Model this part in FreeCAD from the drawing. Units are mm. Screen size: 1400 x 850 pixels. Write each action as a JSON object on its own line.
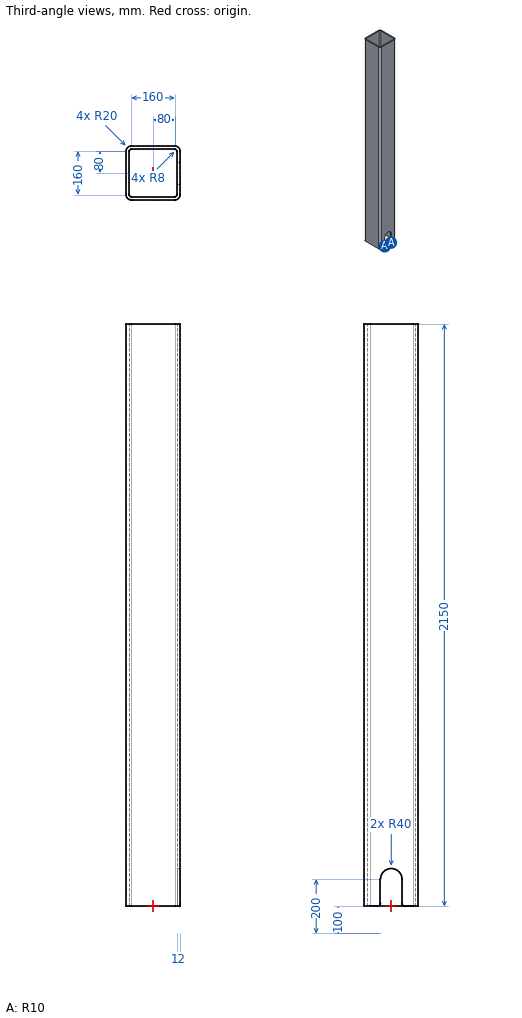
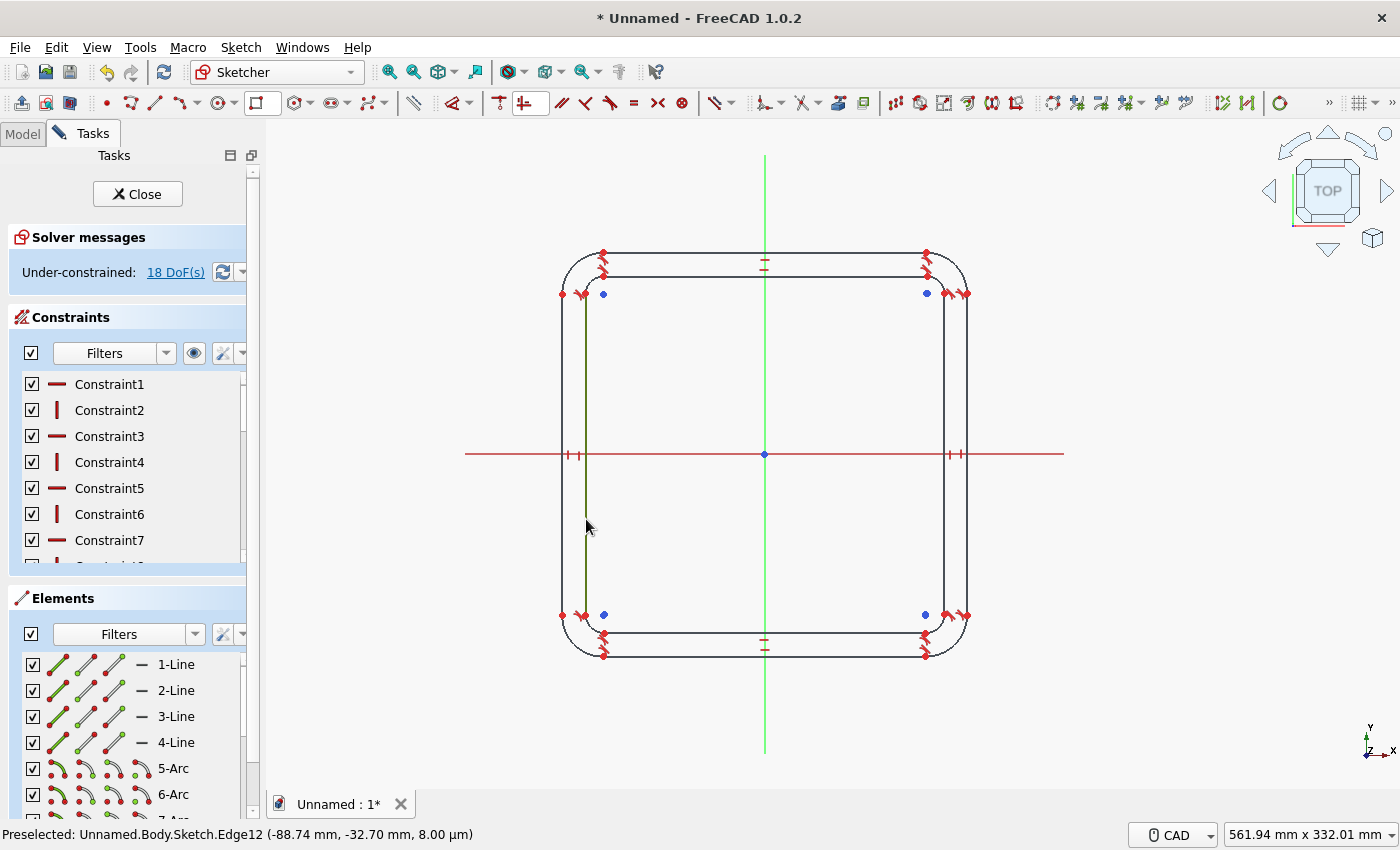
{"action": "left_click", "coordinate": [592, 628]}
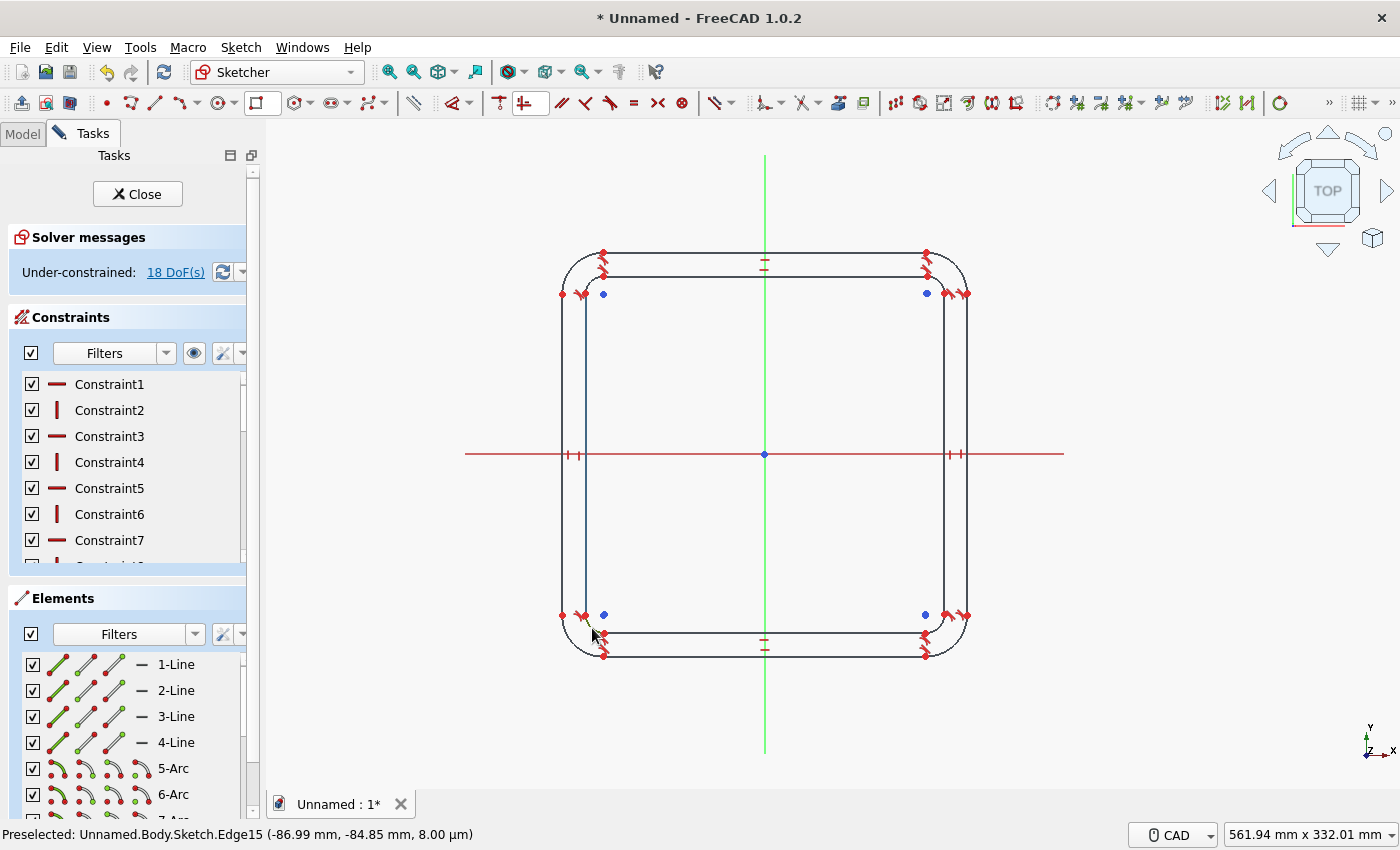
{"action": "left_click", "coordinate": [610, 104]}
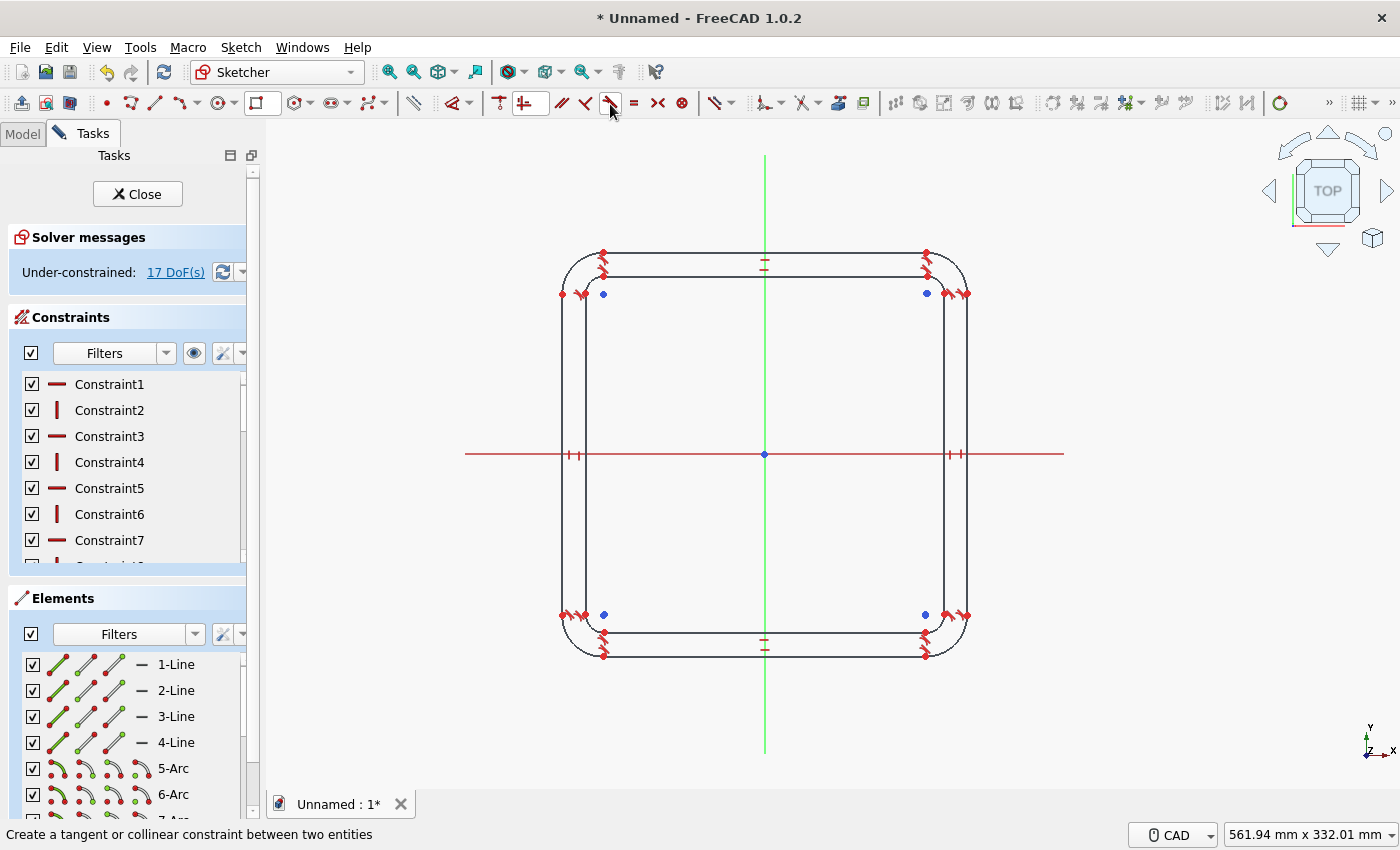
{"action": "left_click", "coordinate": [586, 518]}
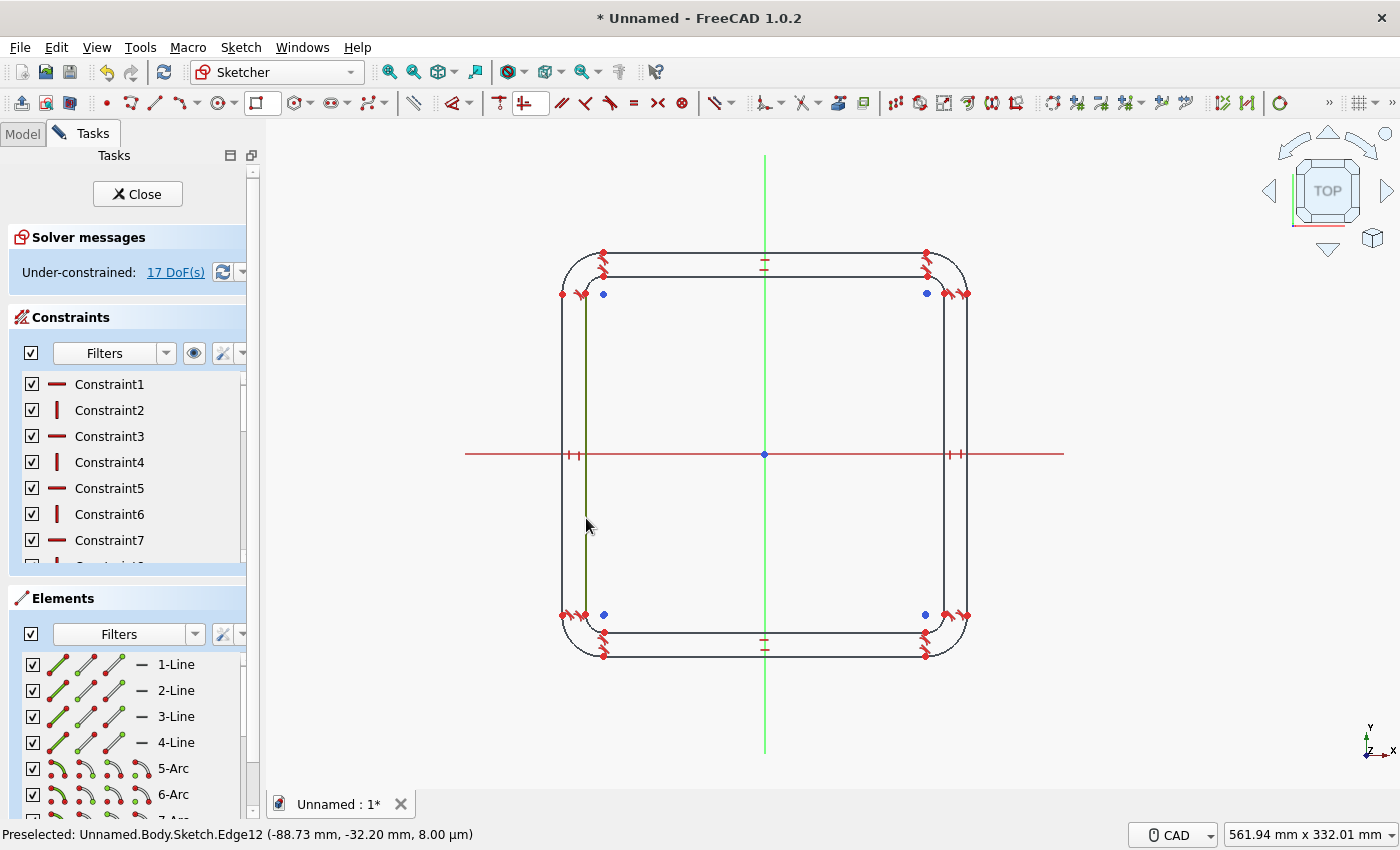
{"action": "left_click", "coordinate": [591, 282]}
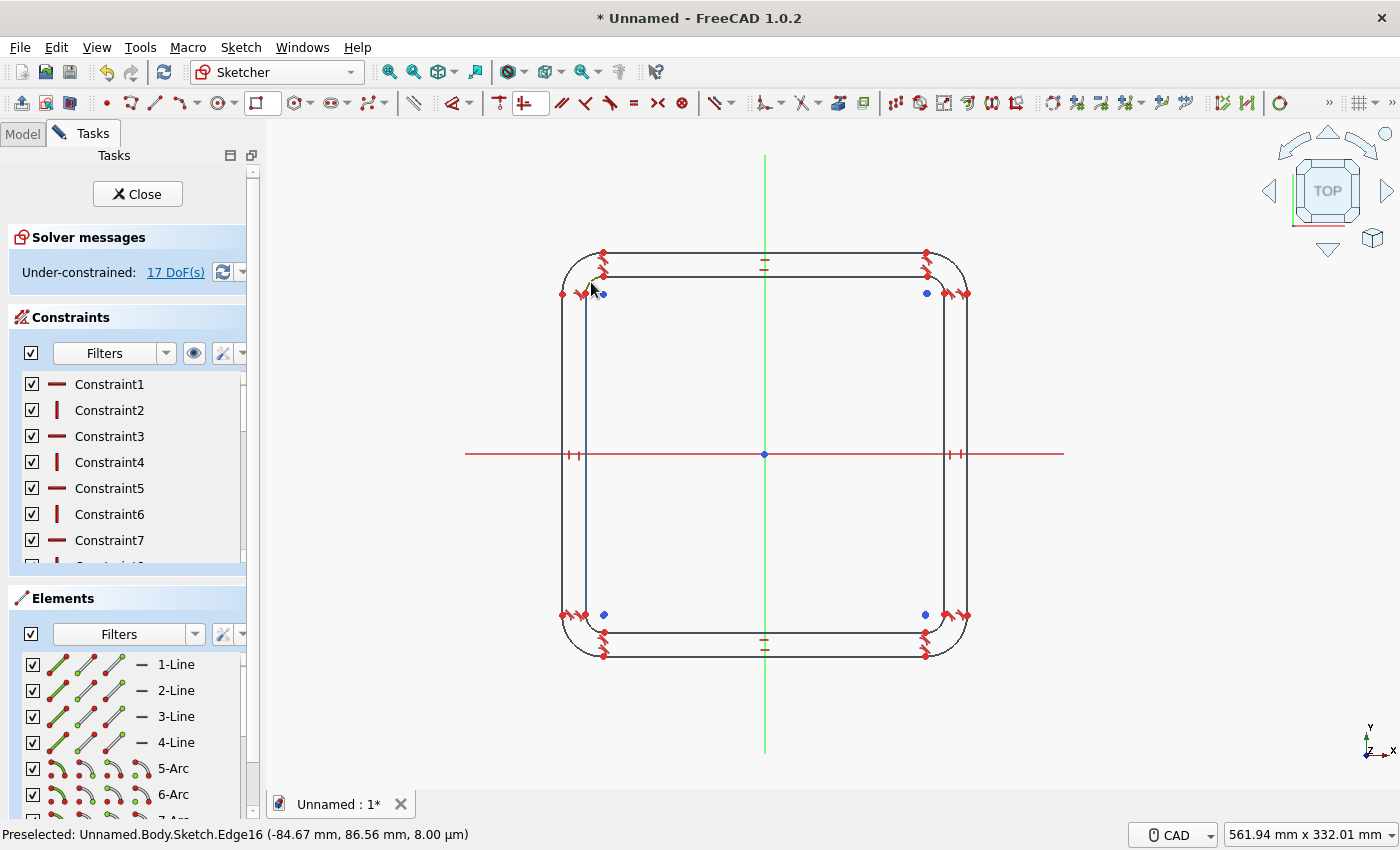
{"action": "left_click", "coordinate": [610, 104]}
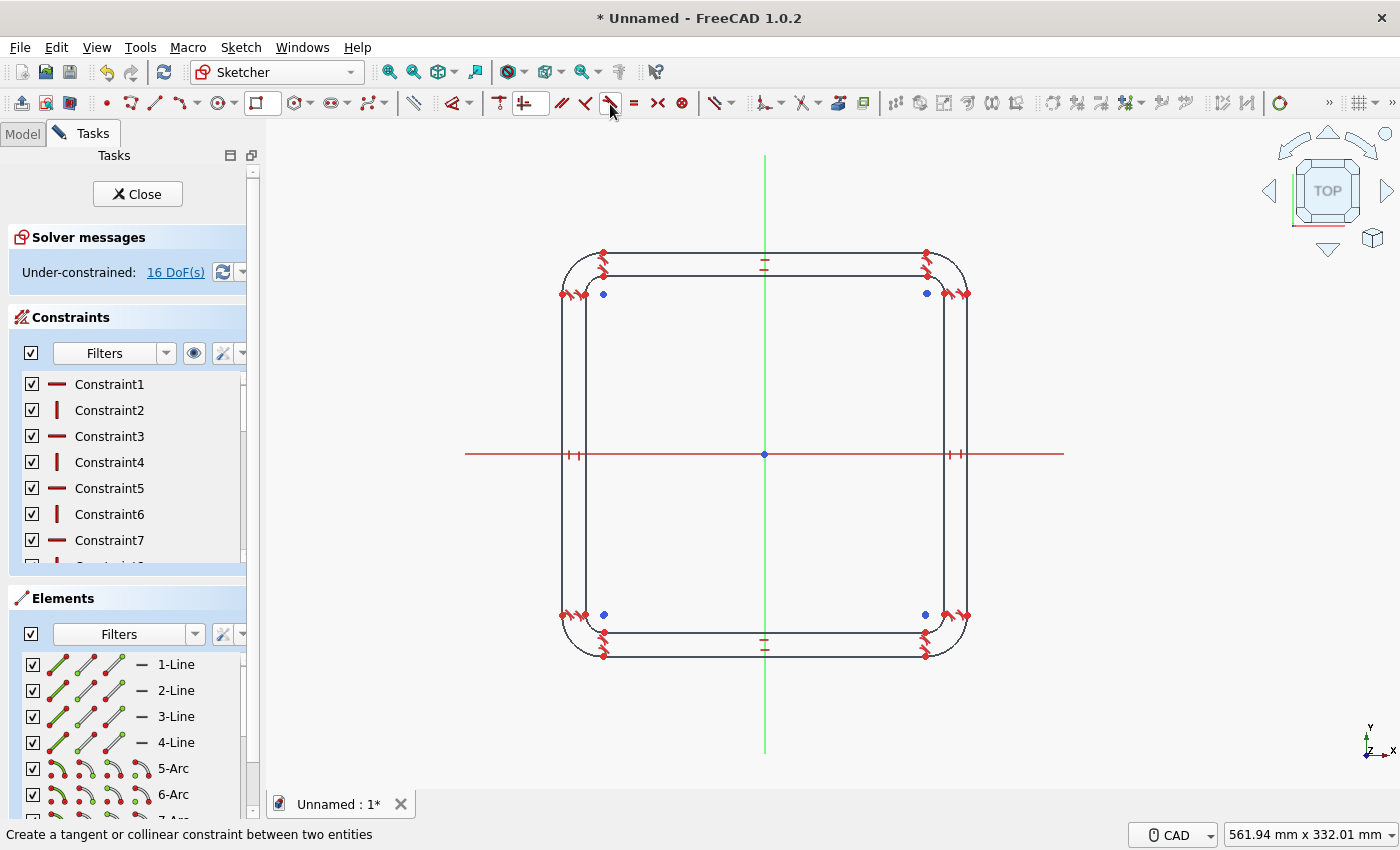
{"action": "left_click", "coordinate": [963, 275]}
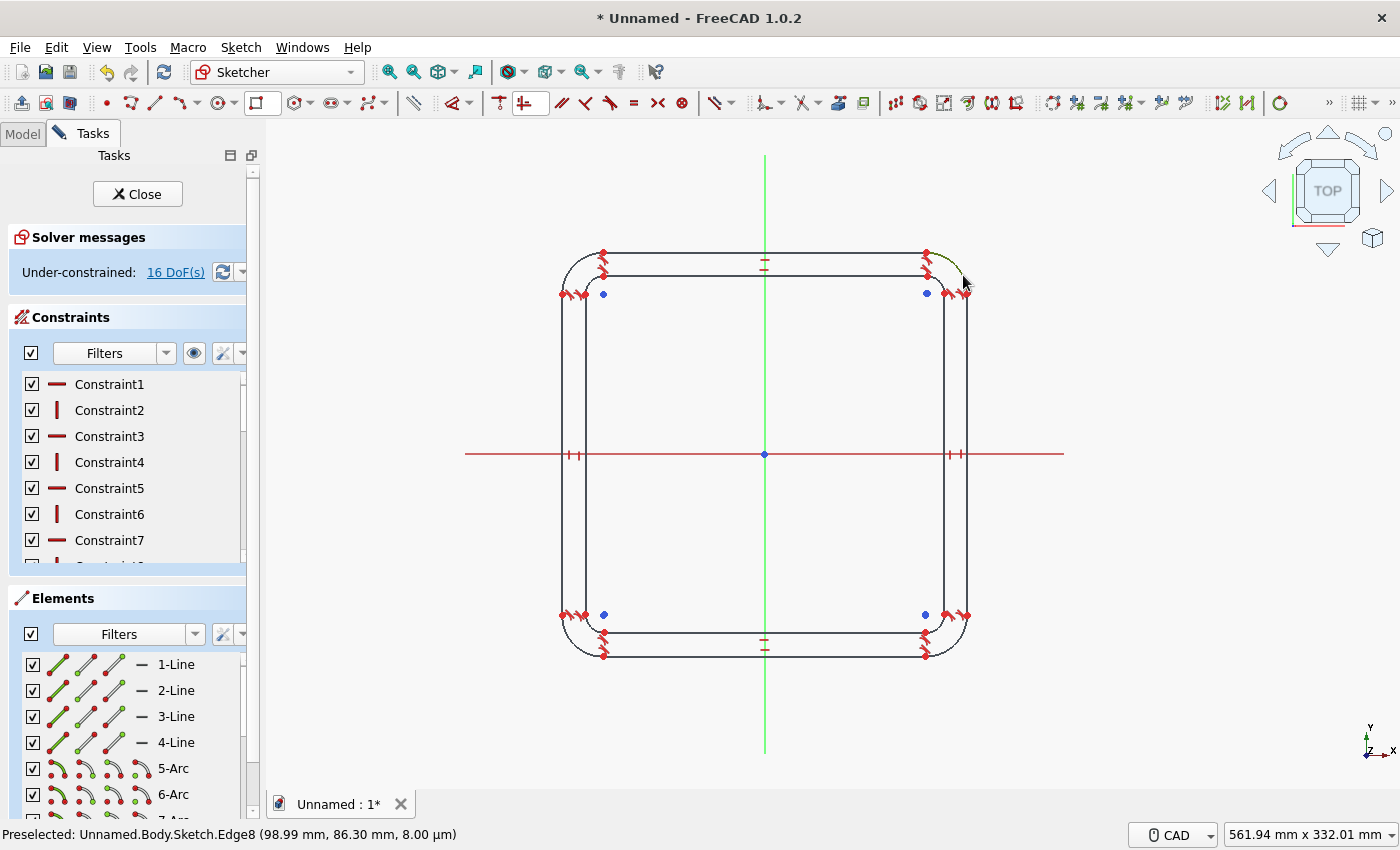
{"action": "left_click", "coordinate": [939, 281]}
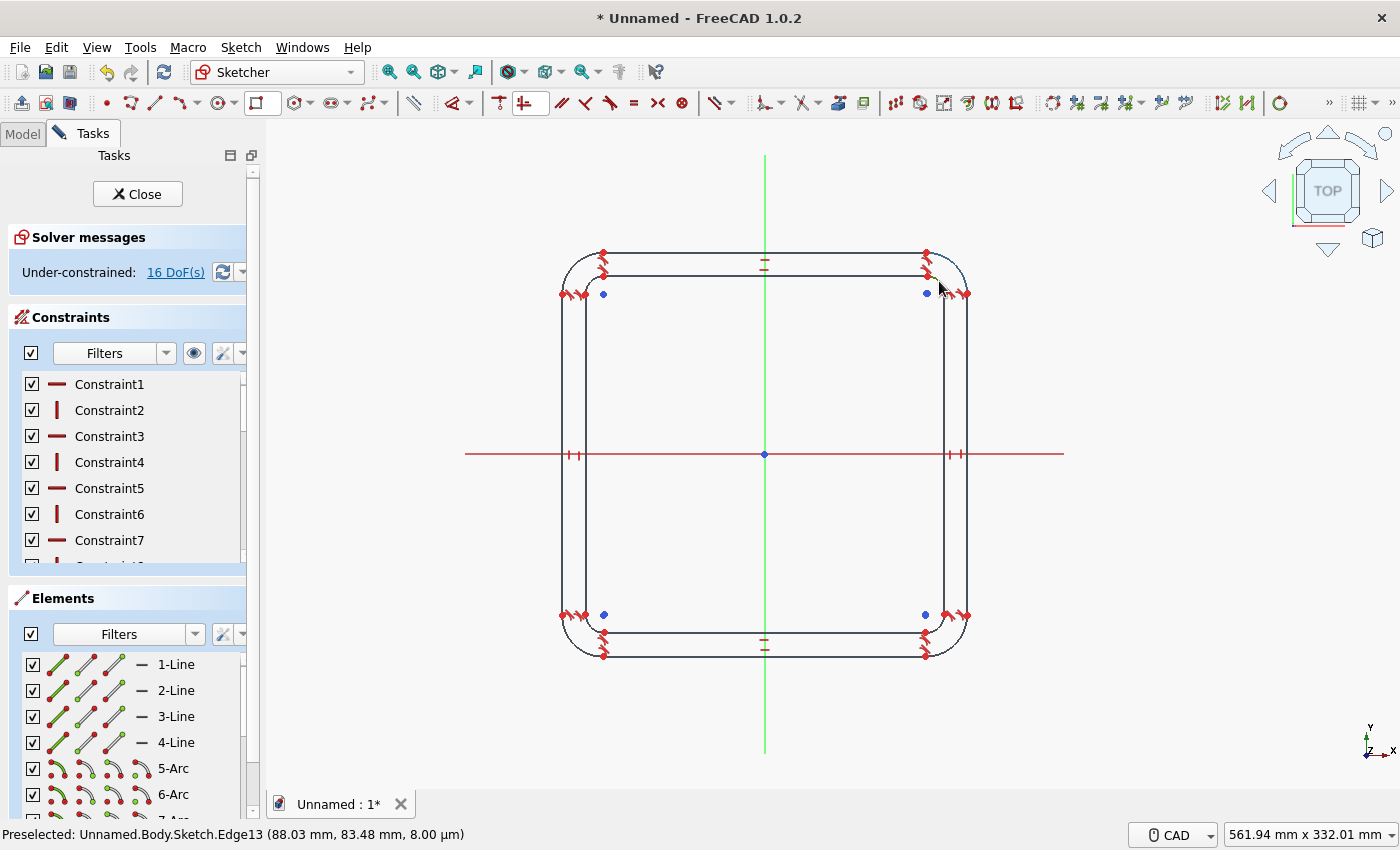
{"action": "left_click", "coordinate": [500, 104]}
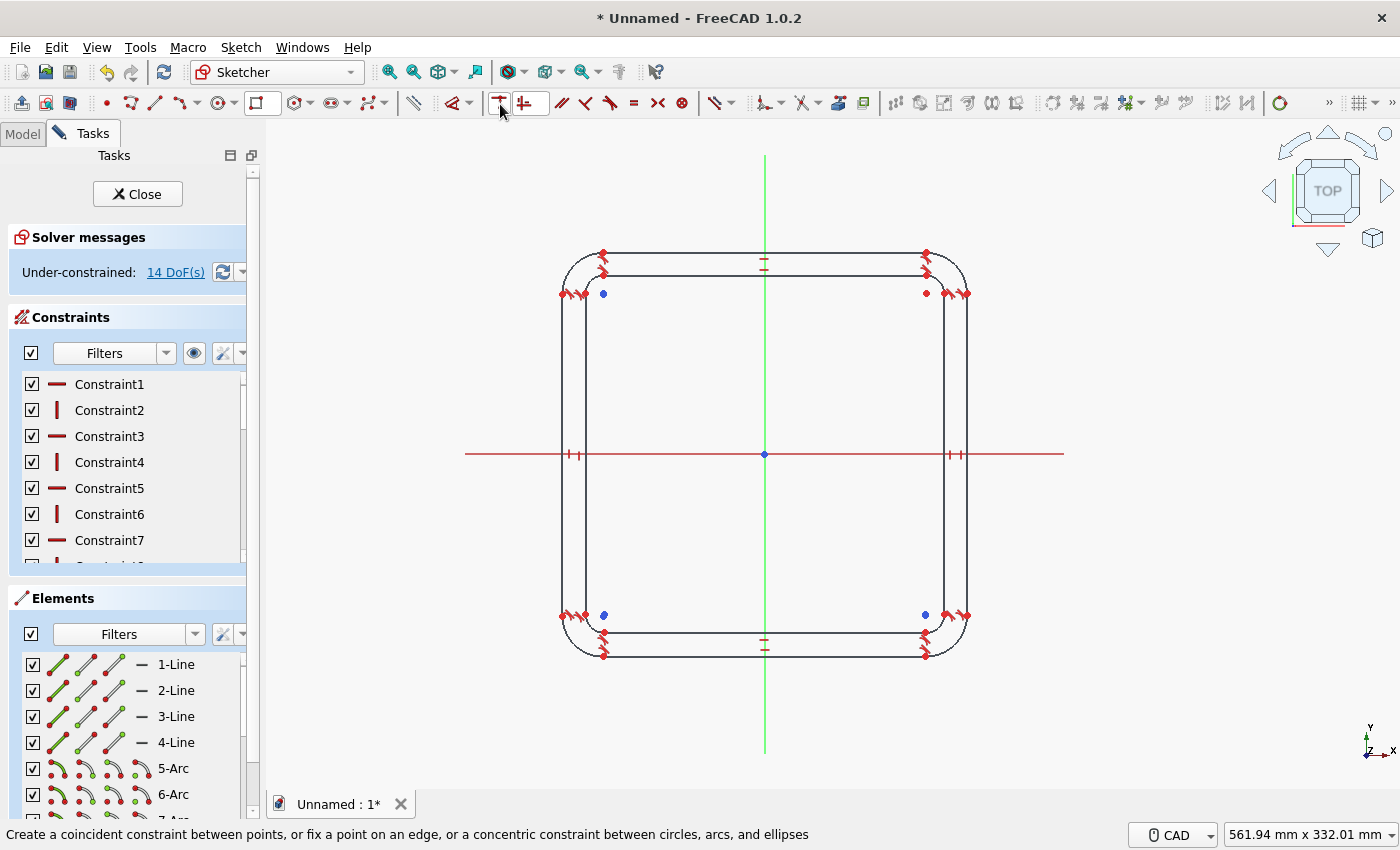
{"action": "left_click", "coordinate": [944, 652]}